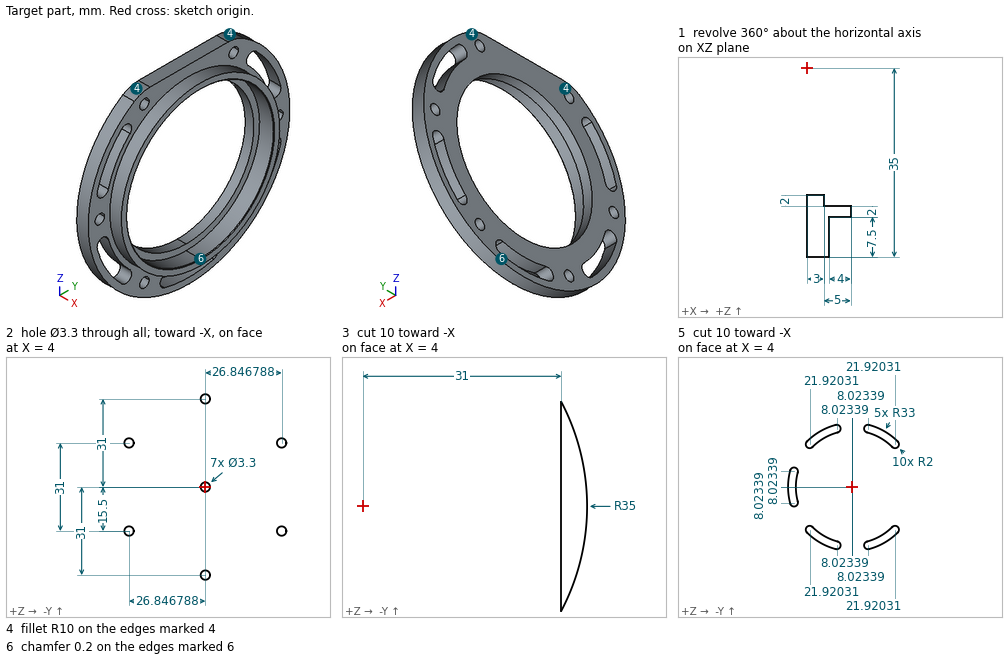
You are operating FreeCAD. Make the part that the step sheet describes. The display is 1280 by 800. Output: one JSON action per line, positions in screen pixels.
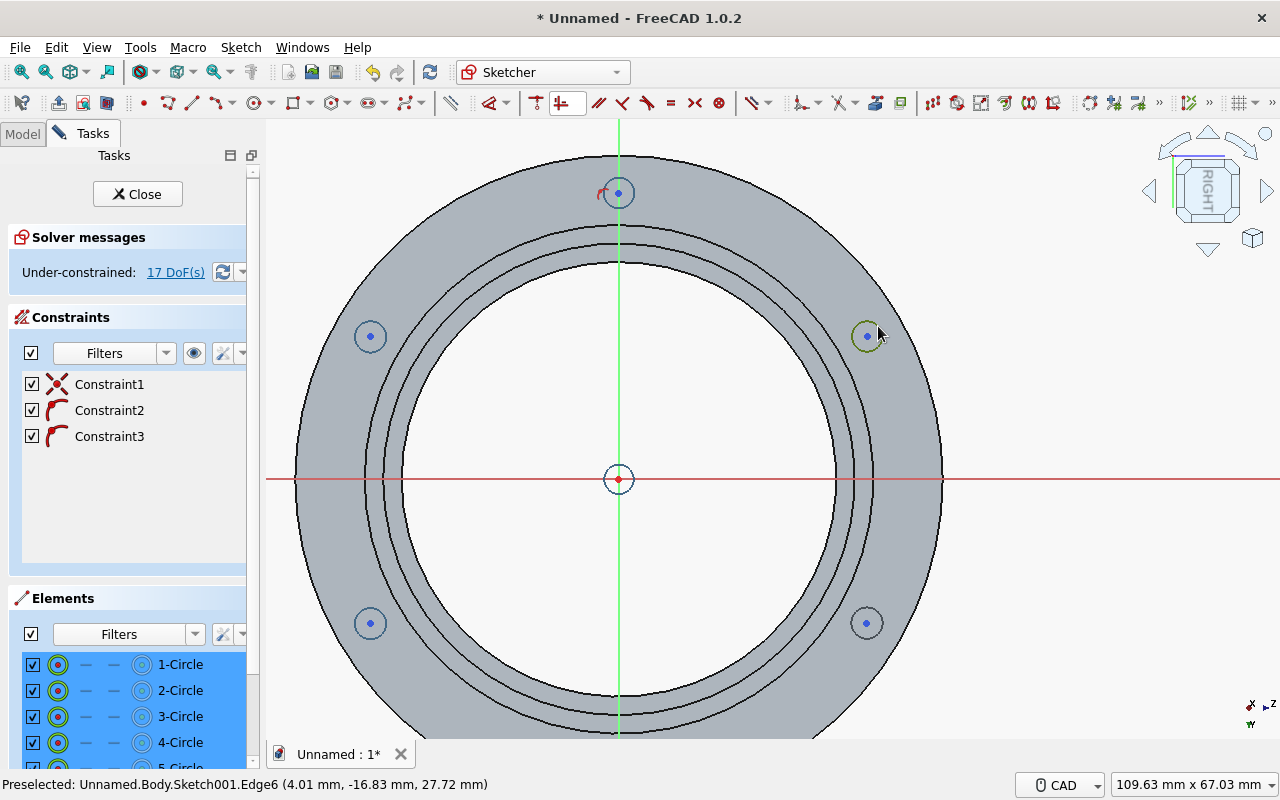
{"action": "left_click", "coordinate": [878, 612]}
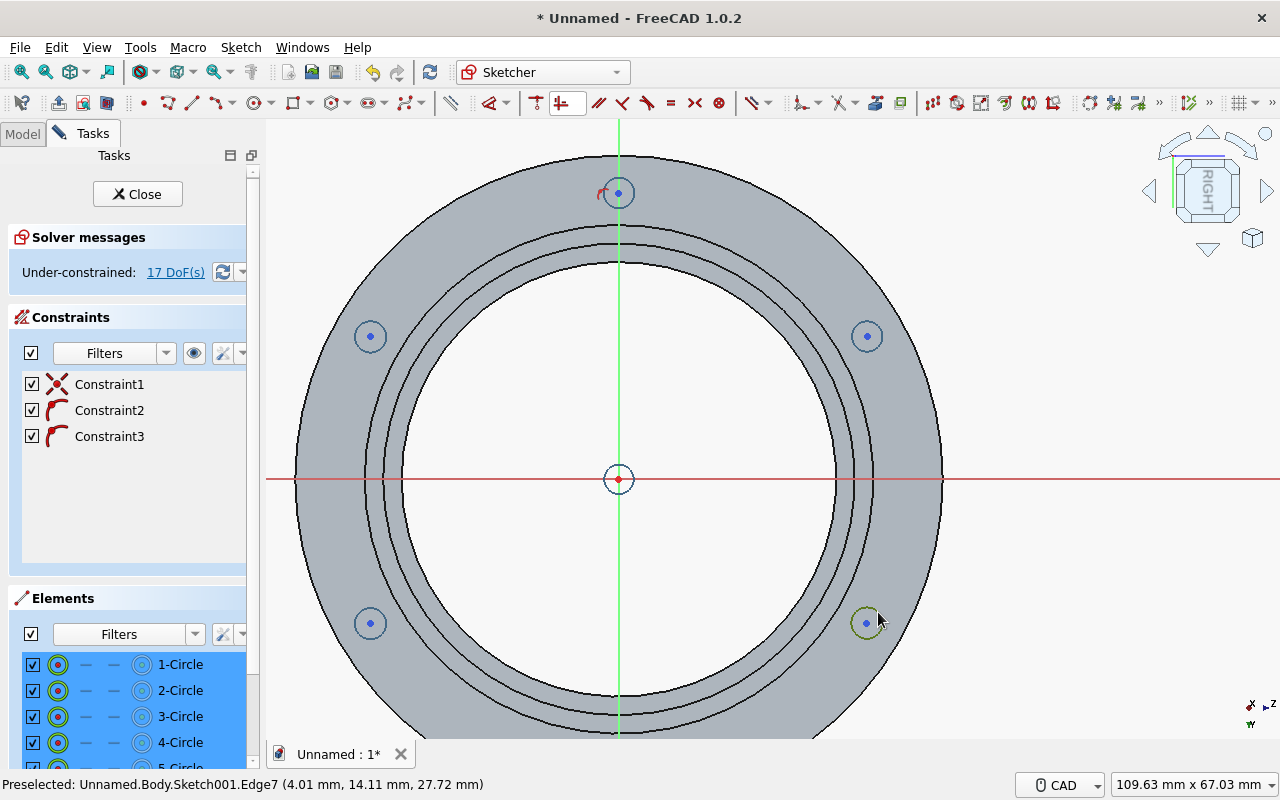
{"action": "left_click", "coordinate": [672, 104]}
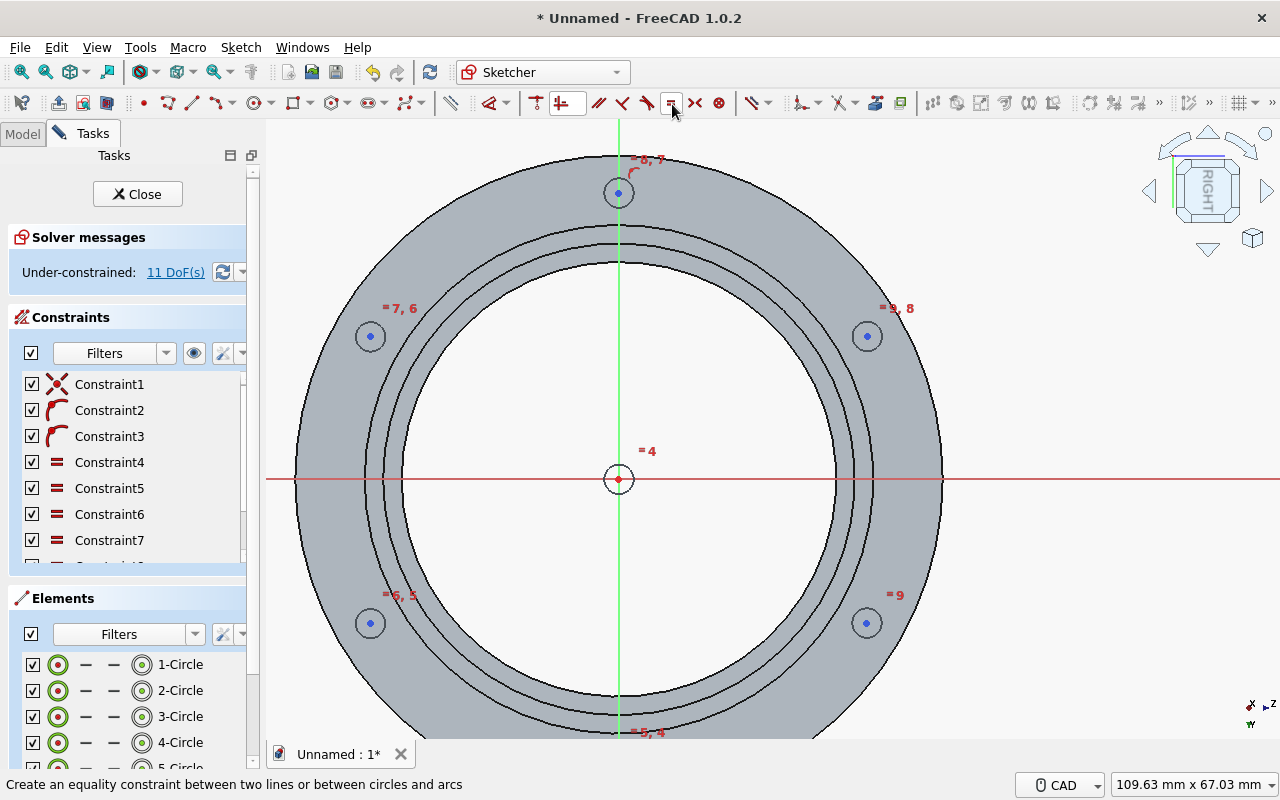
{"action": "left_click", "coordinate": [371, 624]}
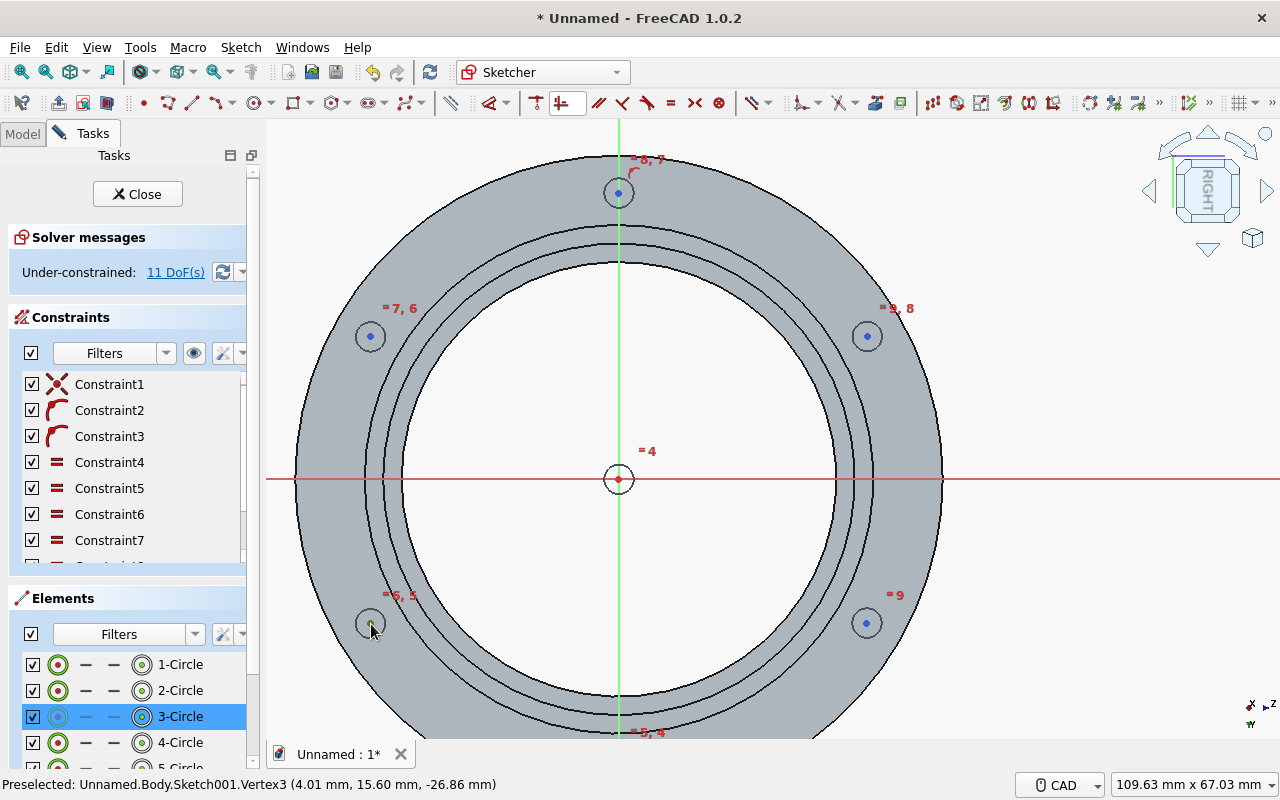
{"action": "left_click", "coordinate": [371, 337]}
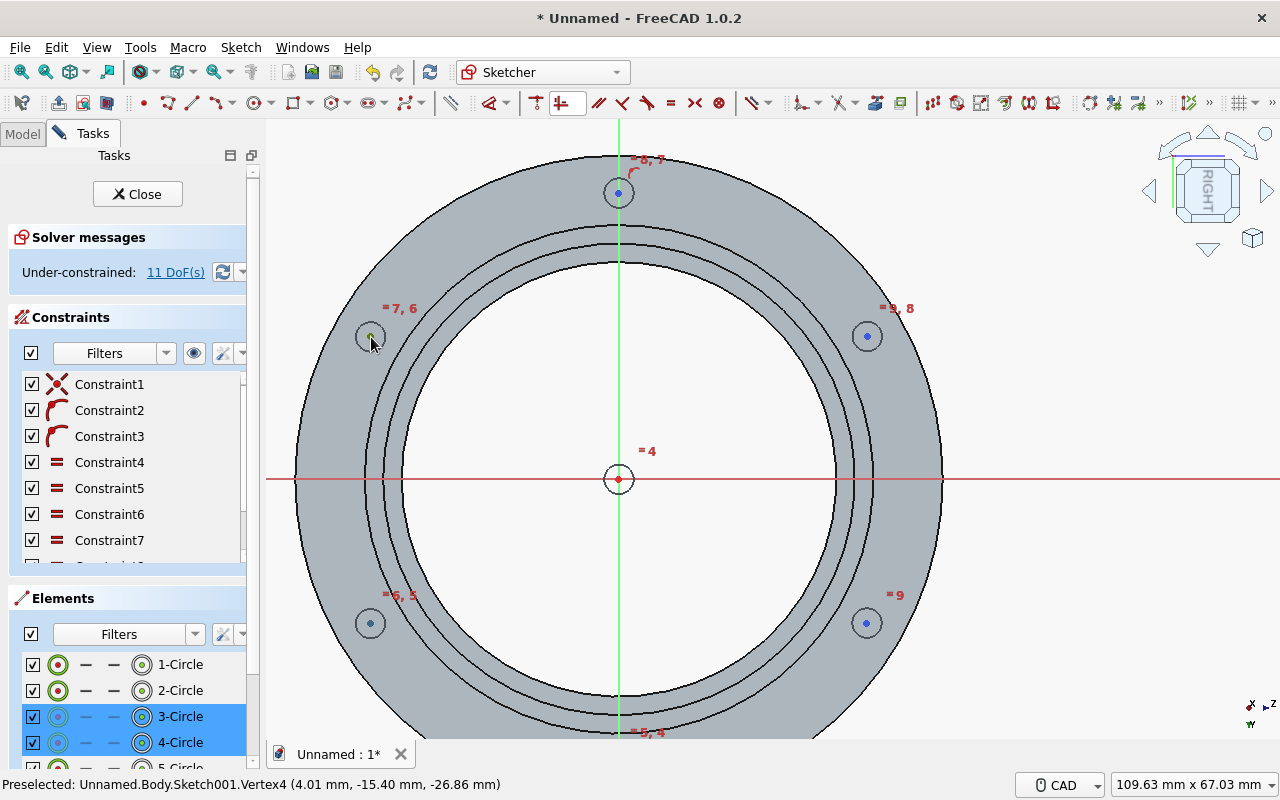
{"action": "key", "text": "v"}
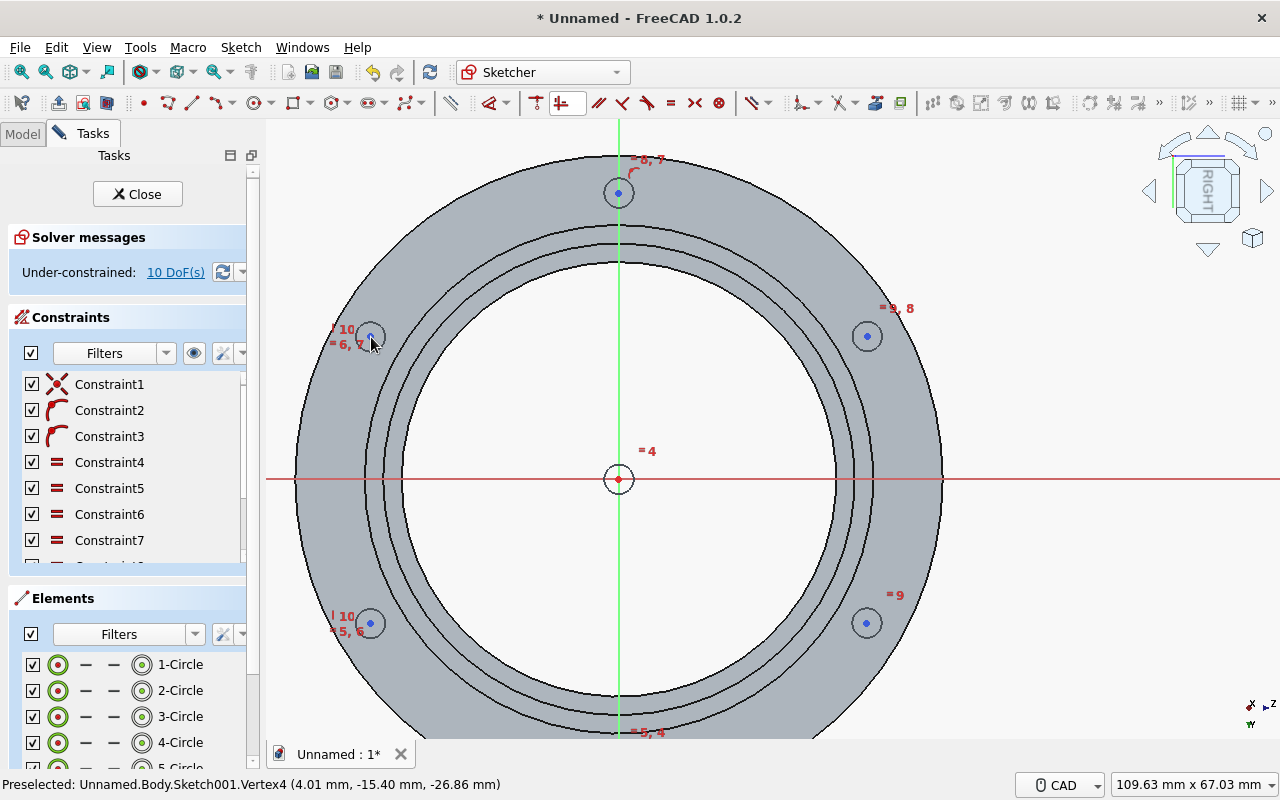
{"action": "left_click", "coordinate": [371, 337]}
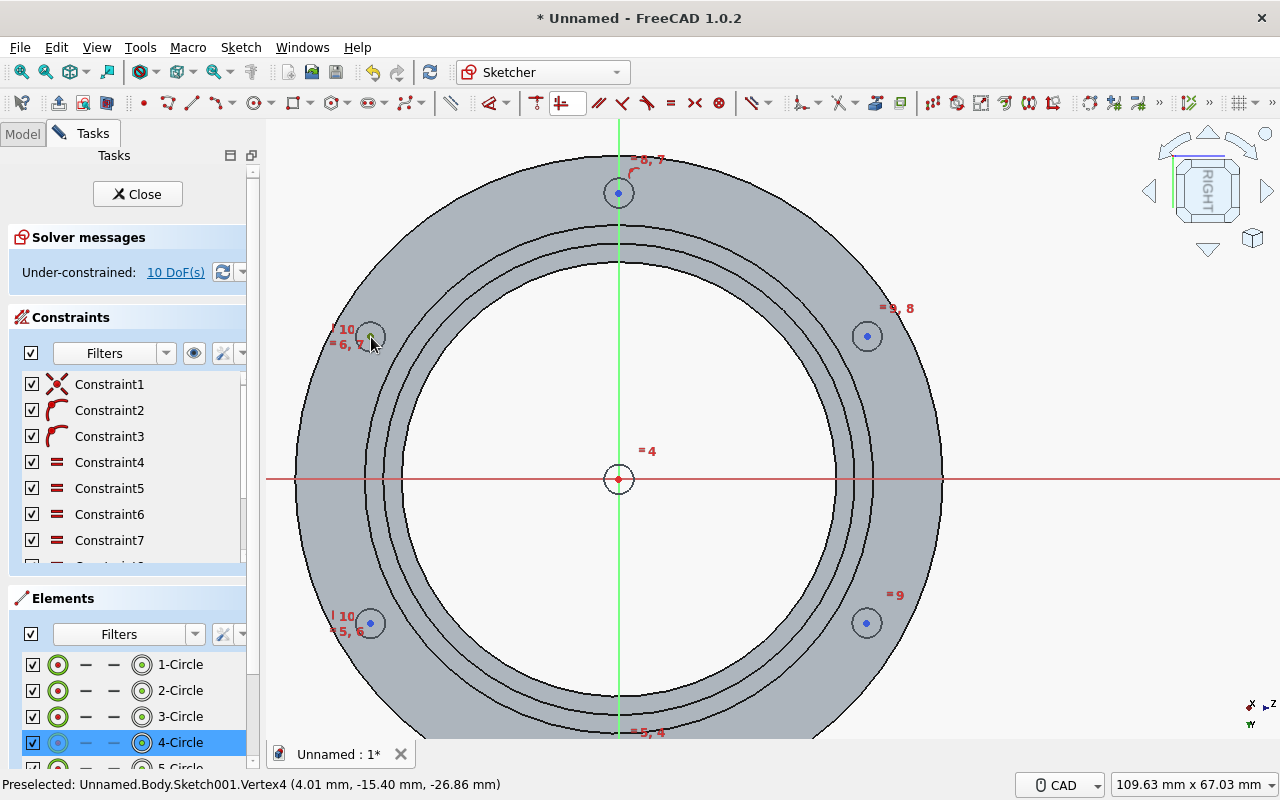
{"action": "left_click", "coordinate": [867, 336]}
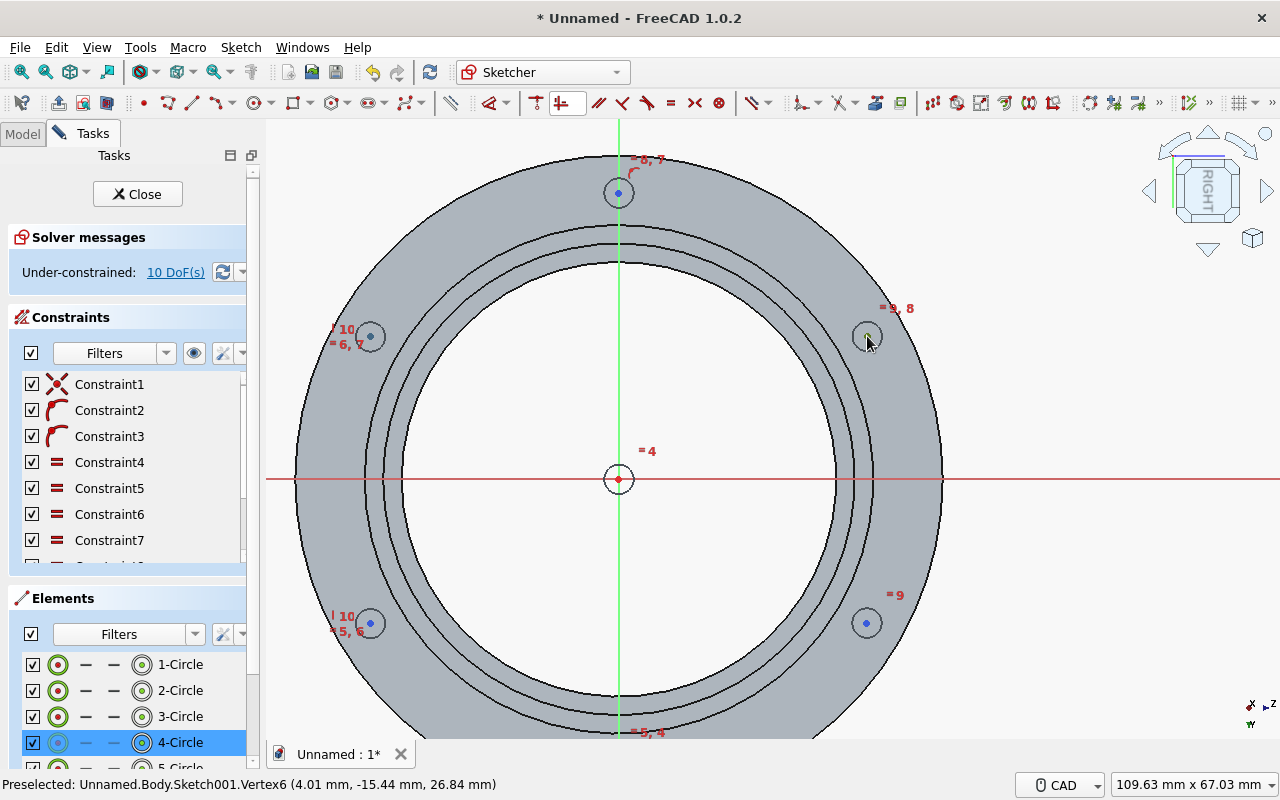
{"action": "left_click", "coordinate": [580, 104]}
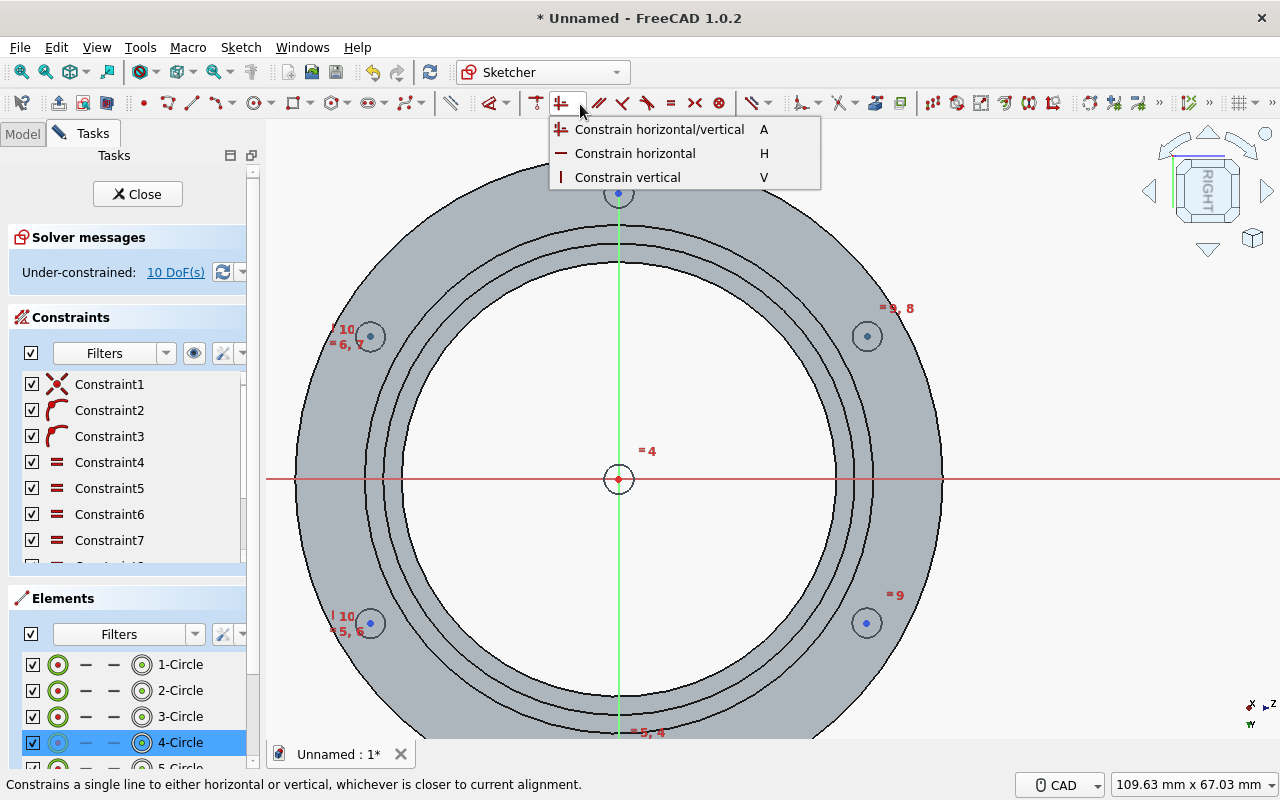
{"action": "left_click", "coordinate": [685, 153]}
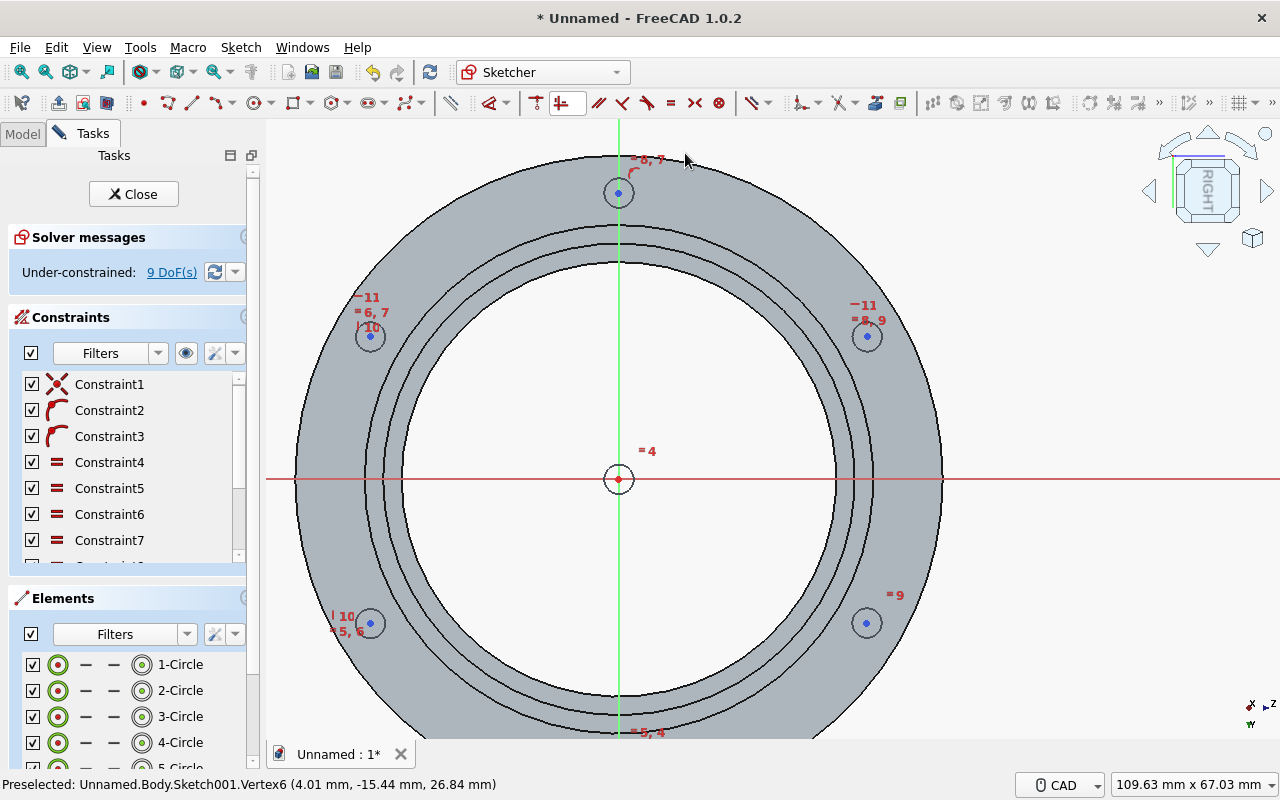
{"action": "left_click", "coordinate": [867, 337]}